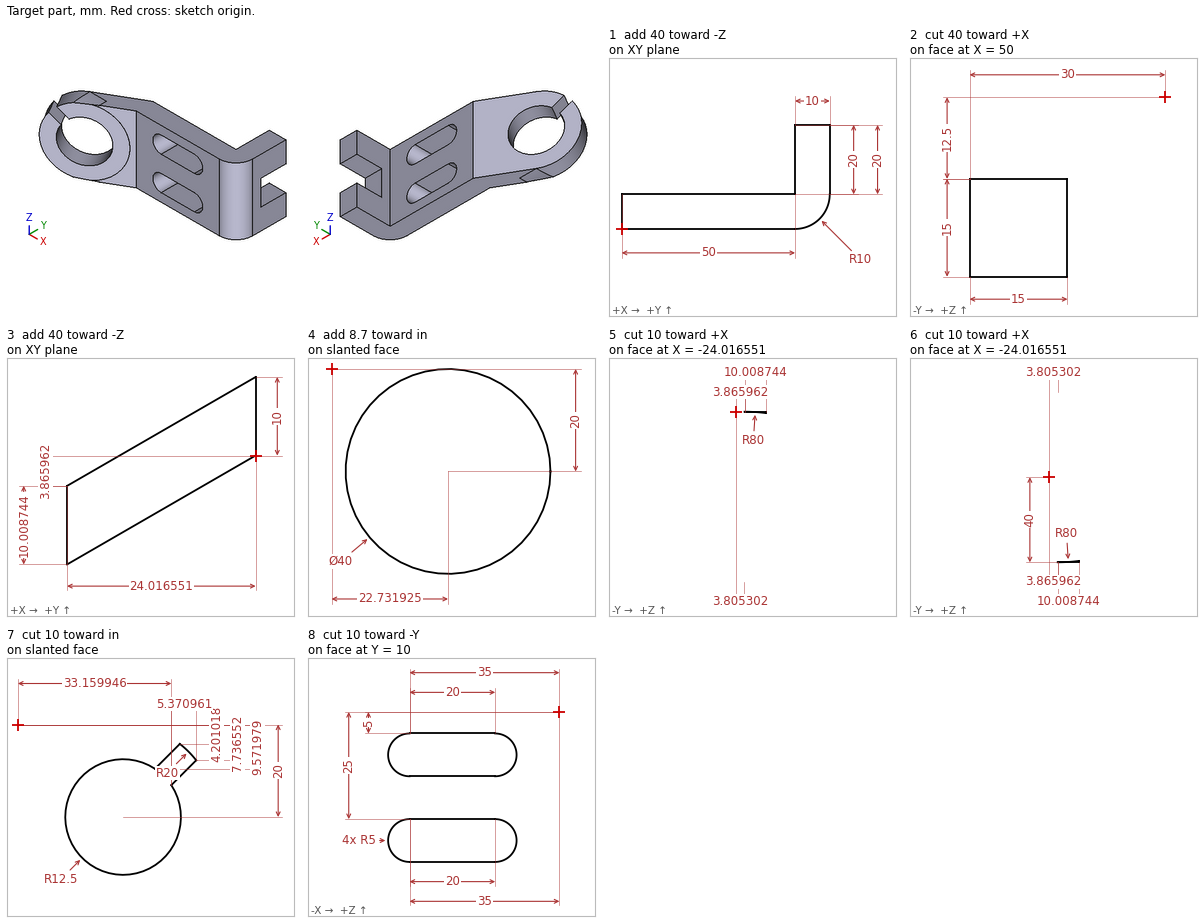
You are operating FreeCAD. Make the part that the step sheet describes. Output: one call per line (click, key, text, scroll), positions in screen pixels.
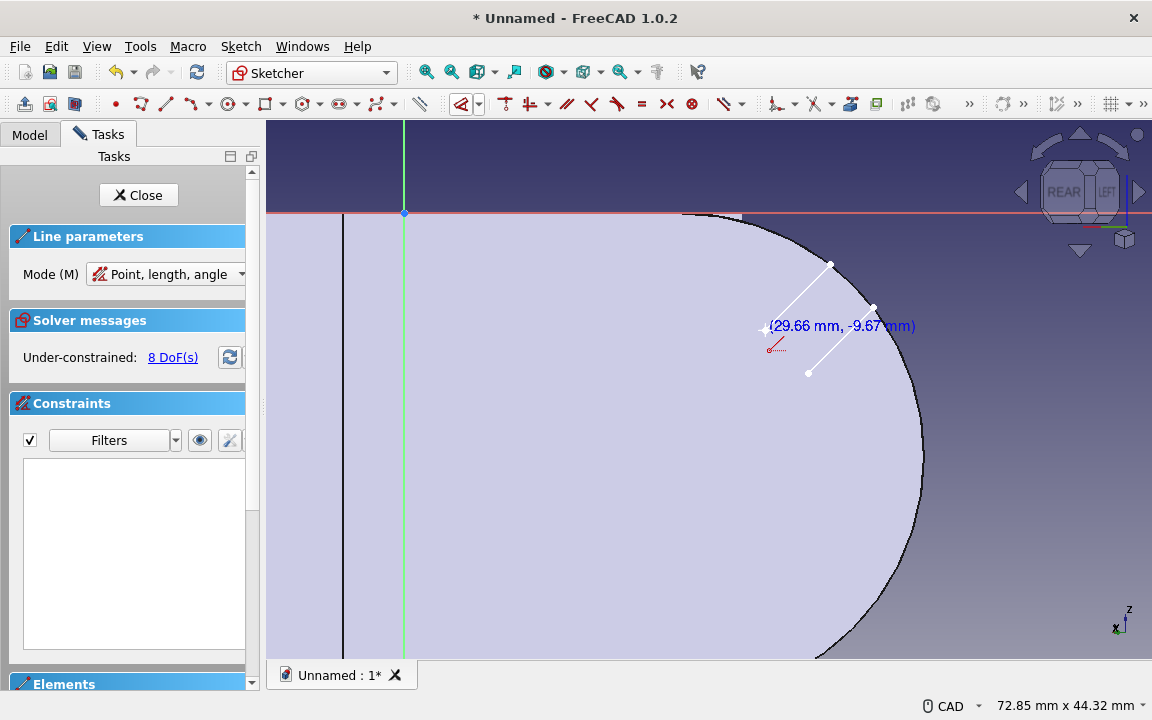
click(190, 104)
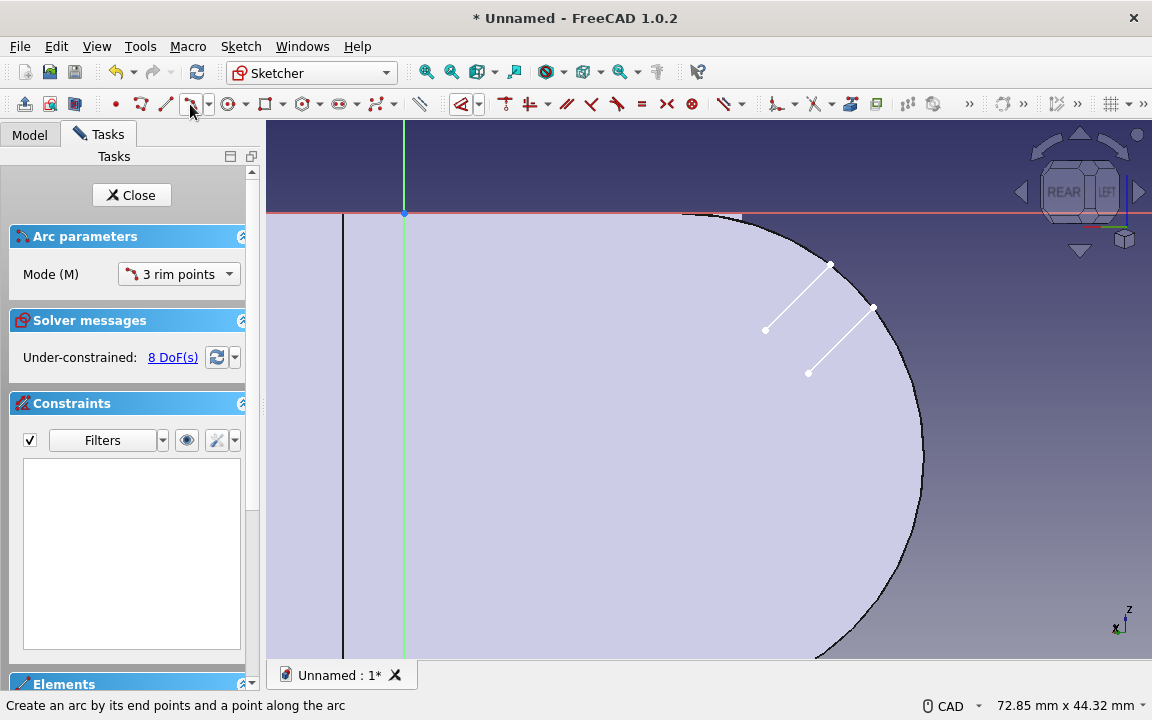
click(873, 308)
click(830, 265)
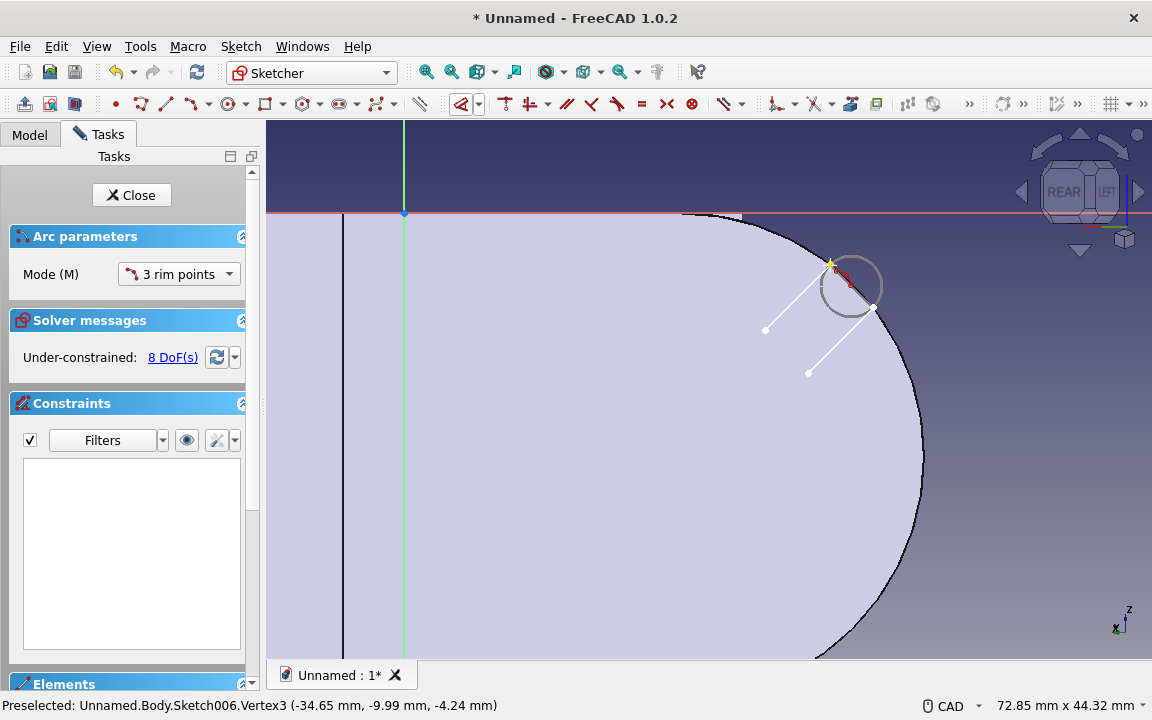
scroll(853, 285, up, 11)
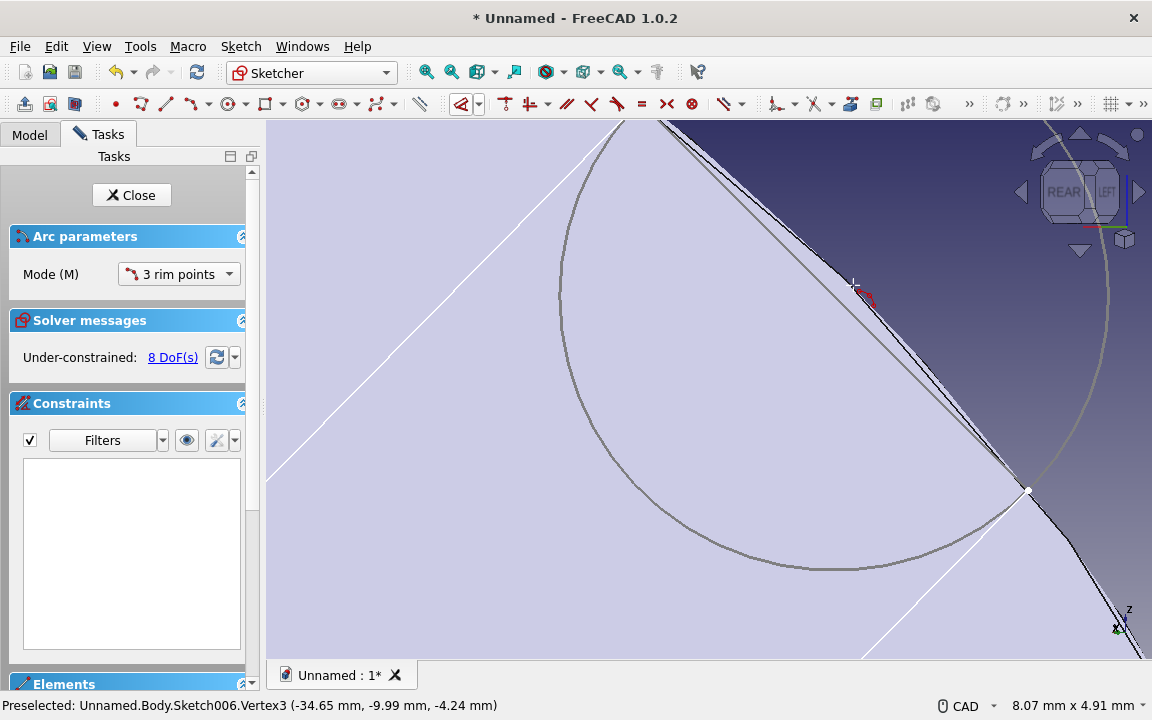
click(845, 279)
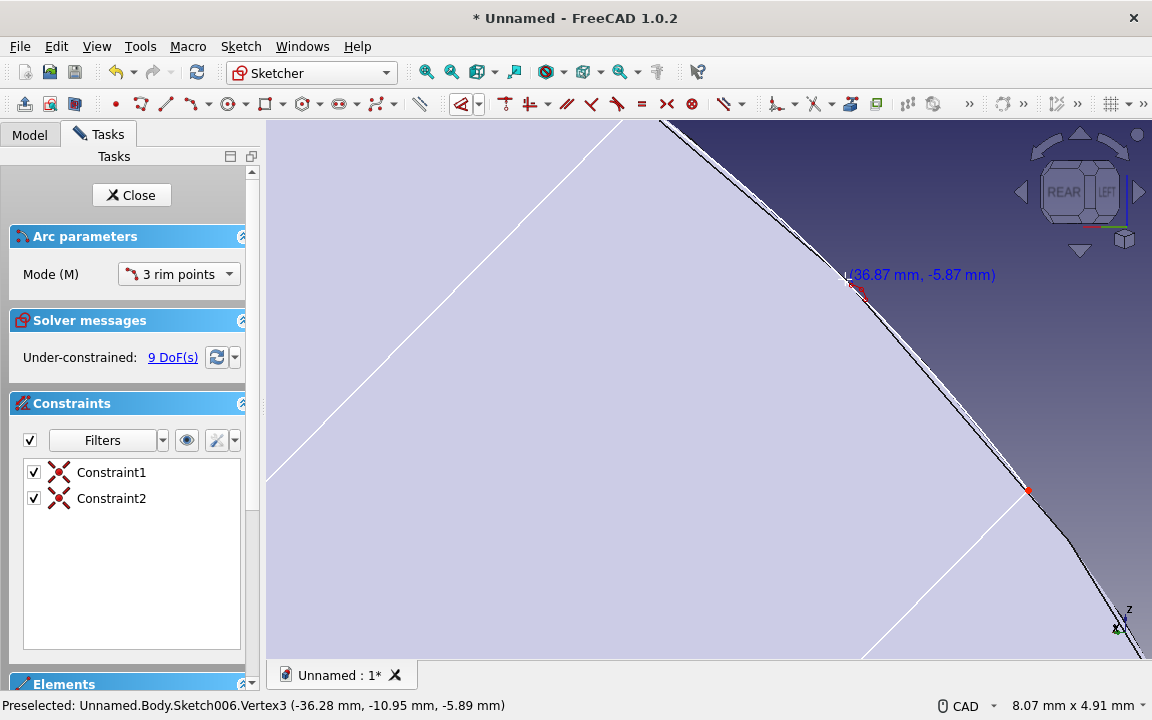
scroll(856, 286, down, 11)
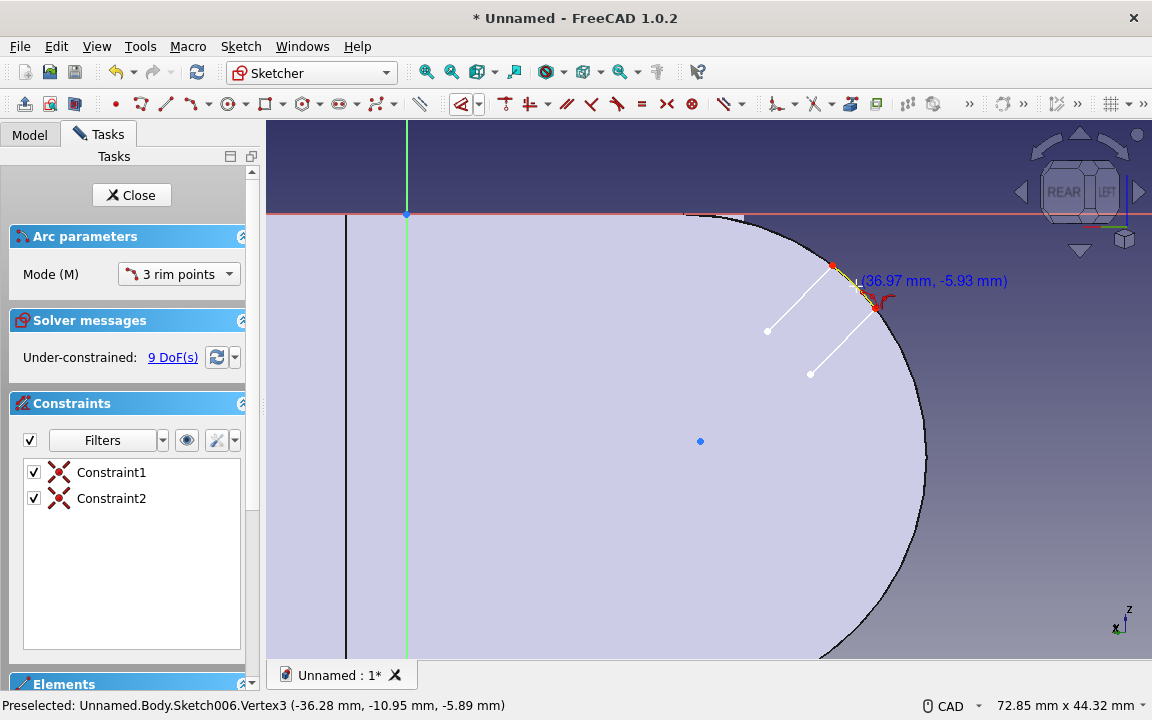
click(768, 332)
click(811, 375)
click(576, 565)
key(Escape)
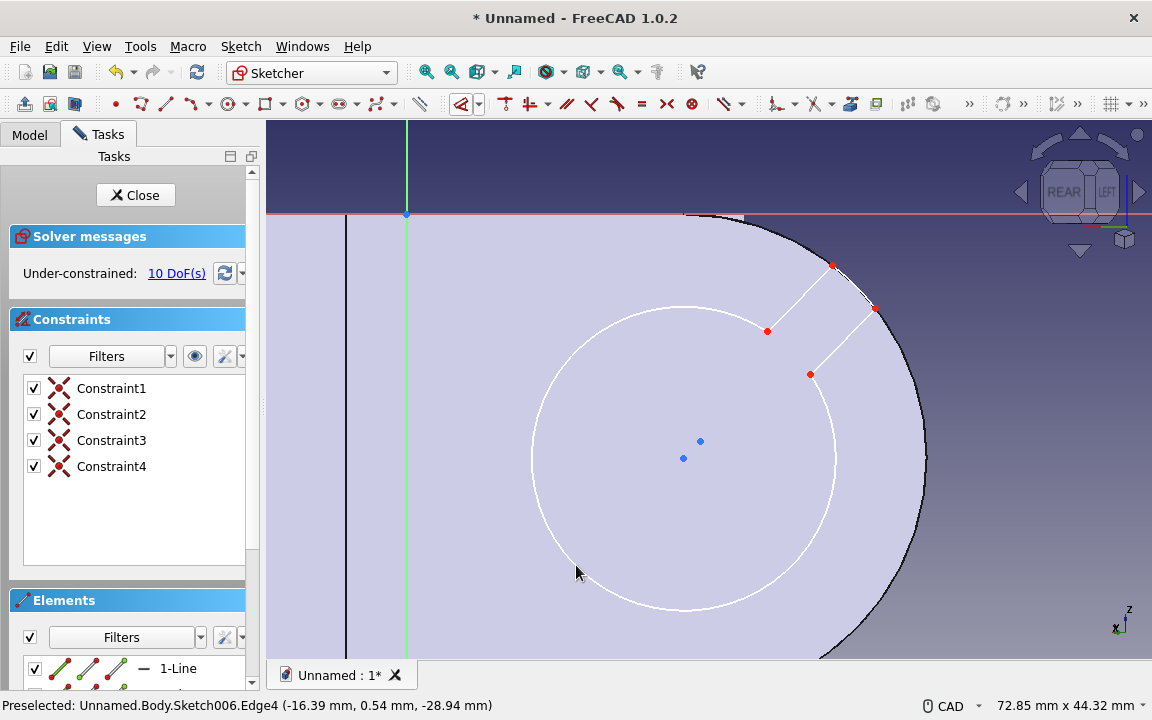
click(864, 295)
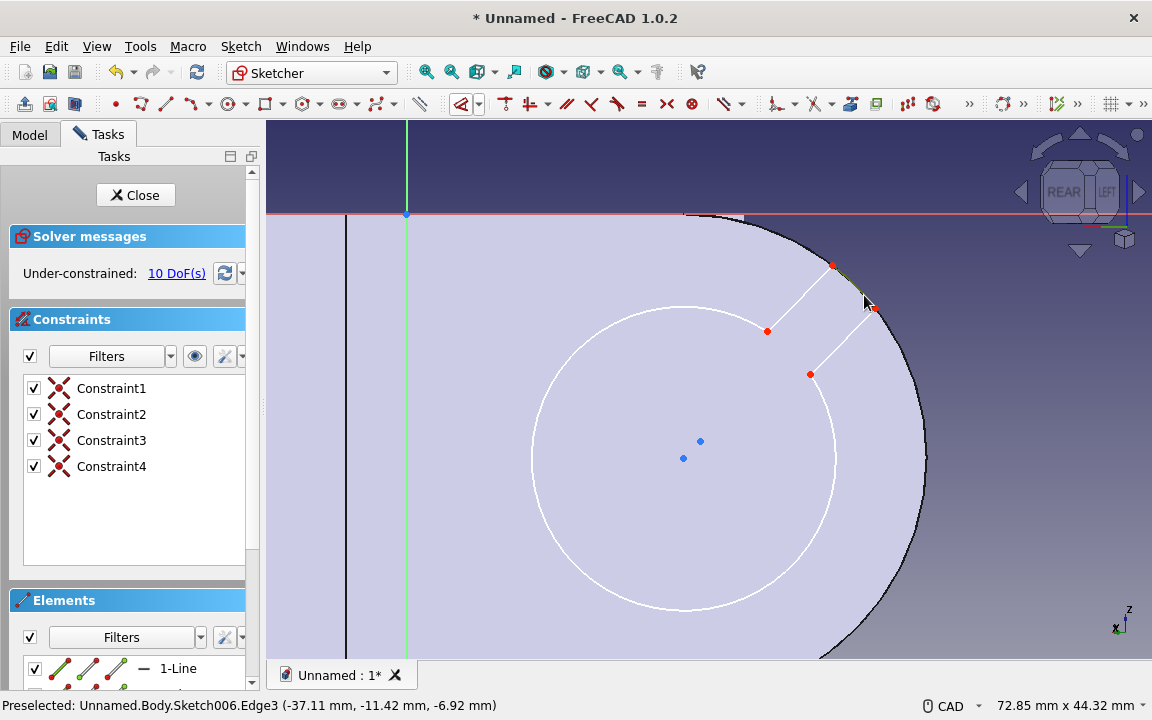
click(543, 401)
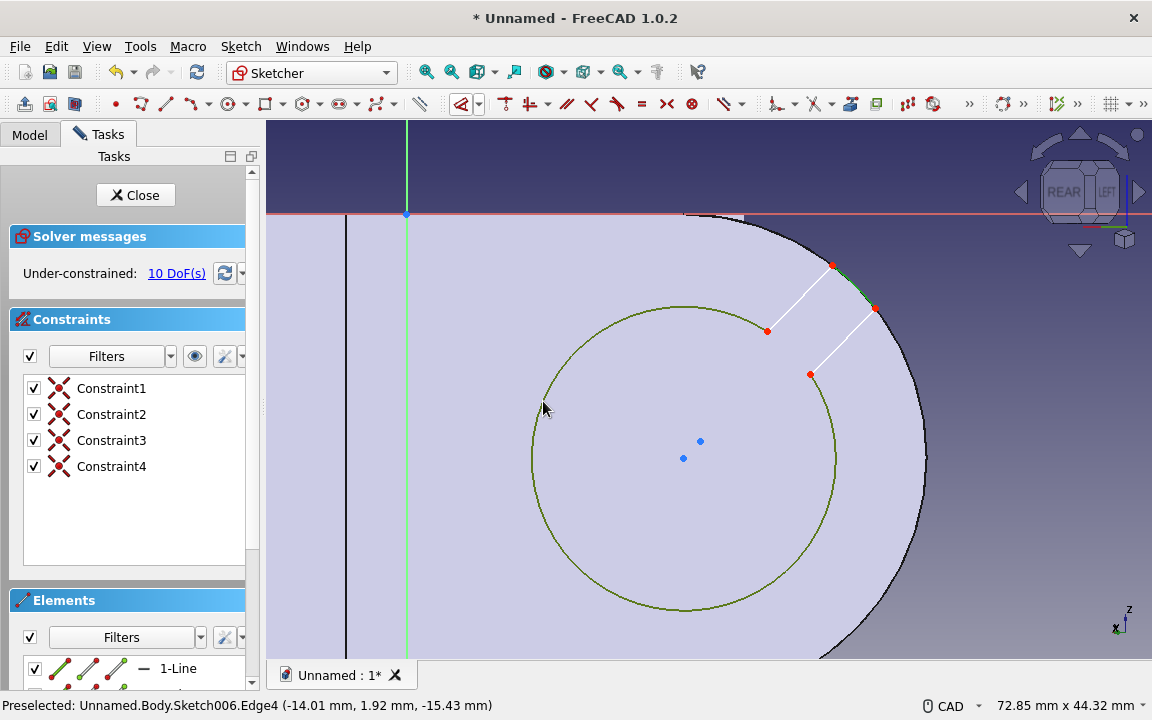
click(505, 104)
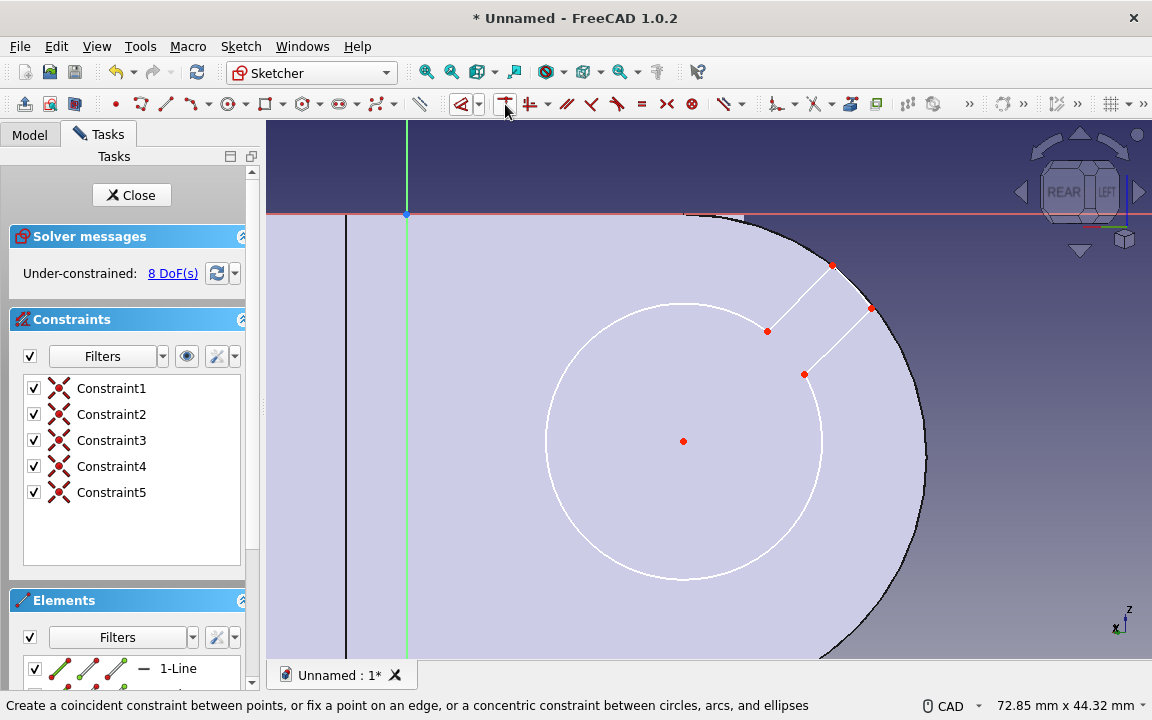
click(861, 295)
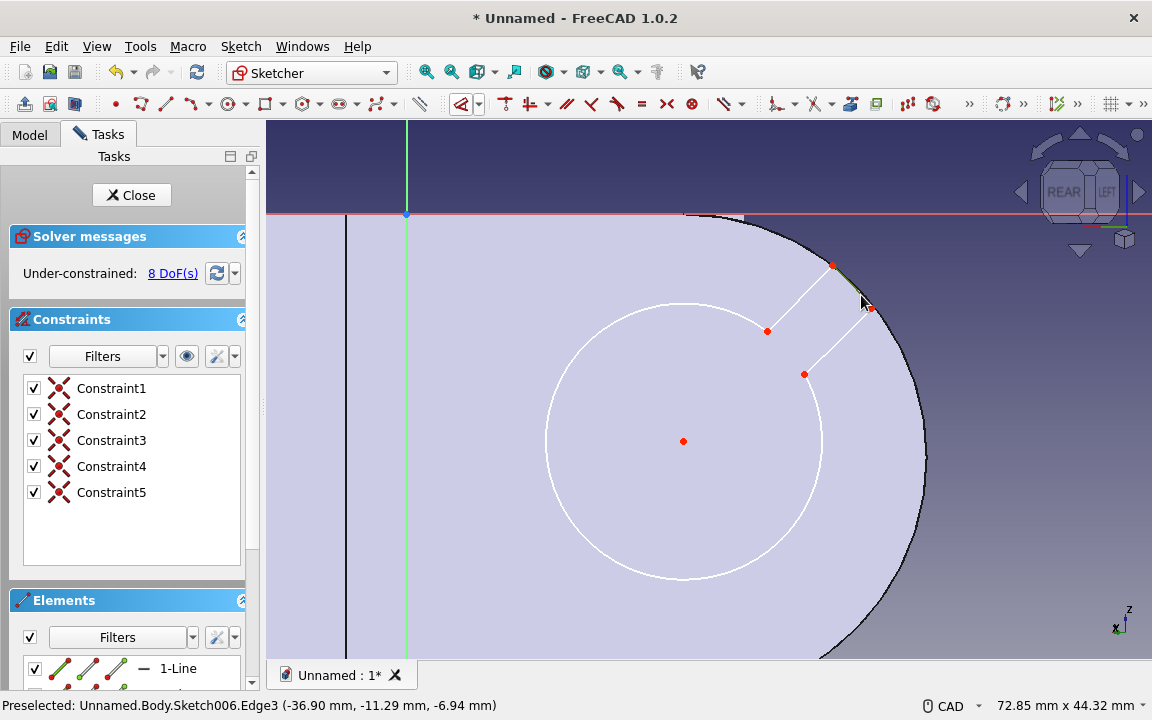
click(478, 104)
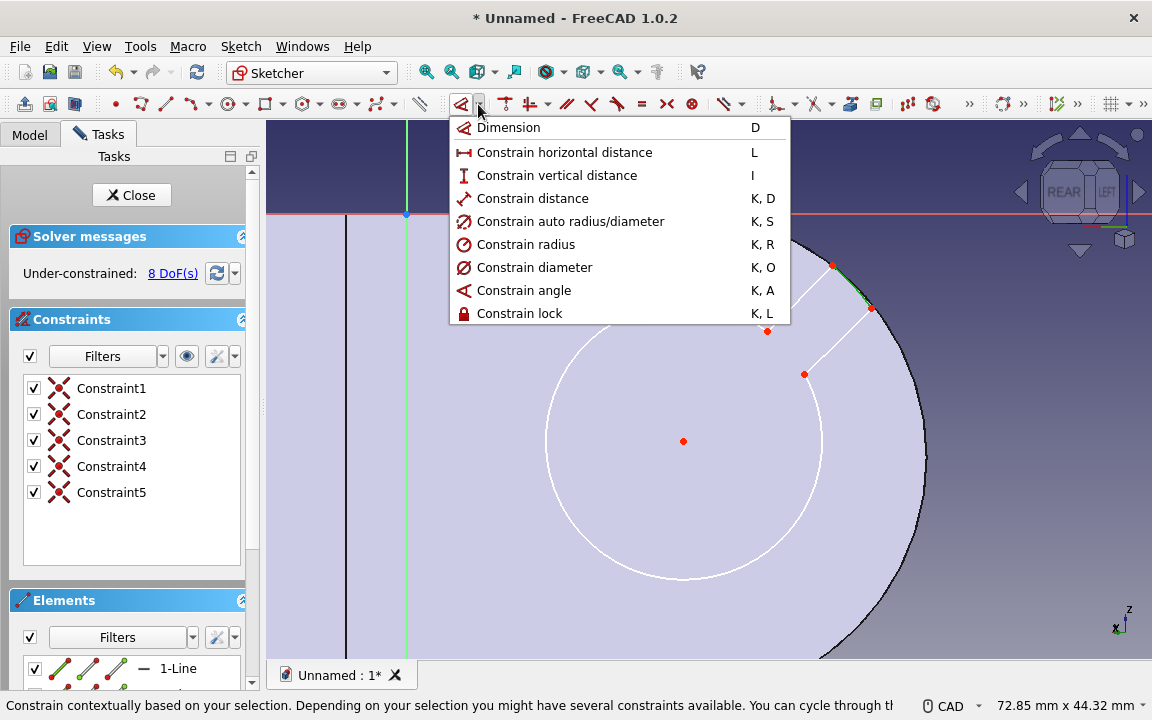
click(620, 244)